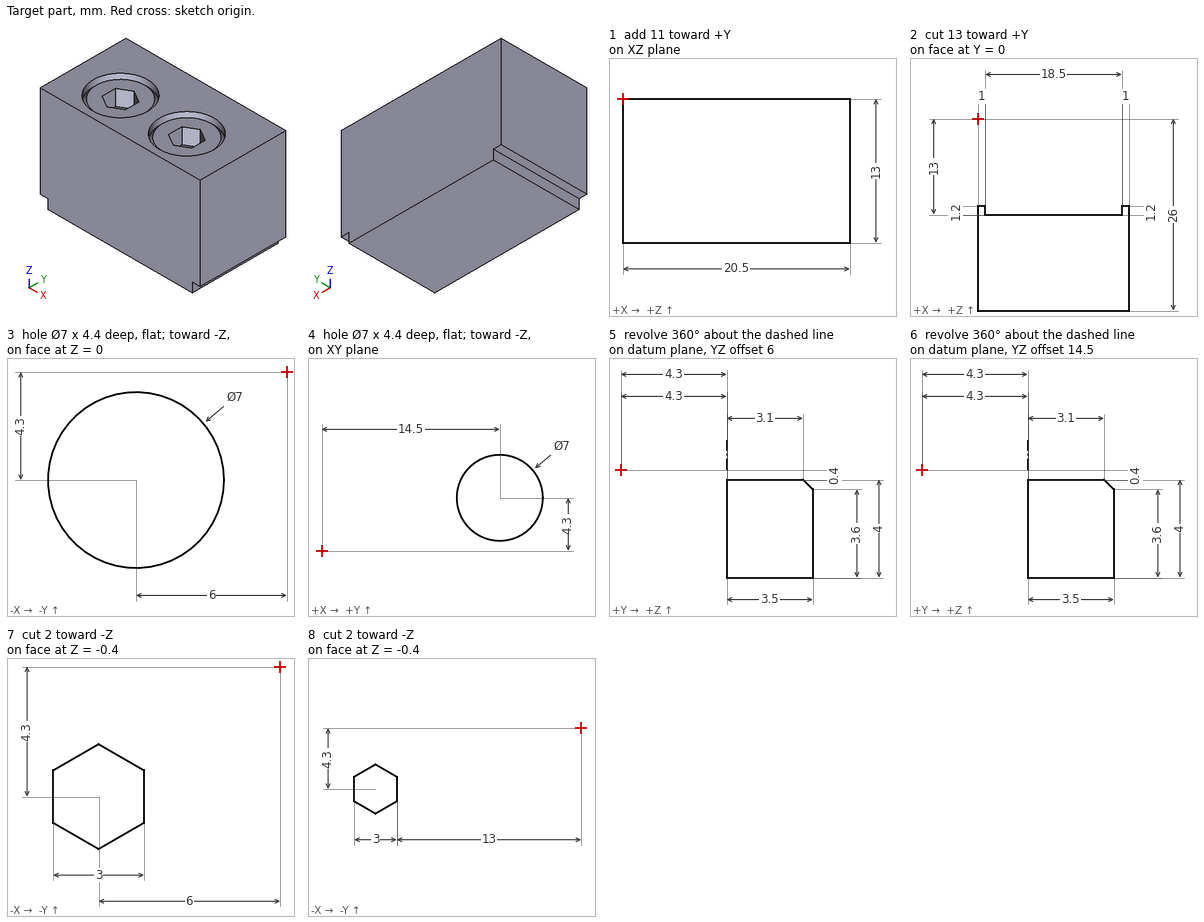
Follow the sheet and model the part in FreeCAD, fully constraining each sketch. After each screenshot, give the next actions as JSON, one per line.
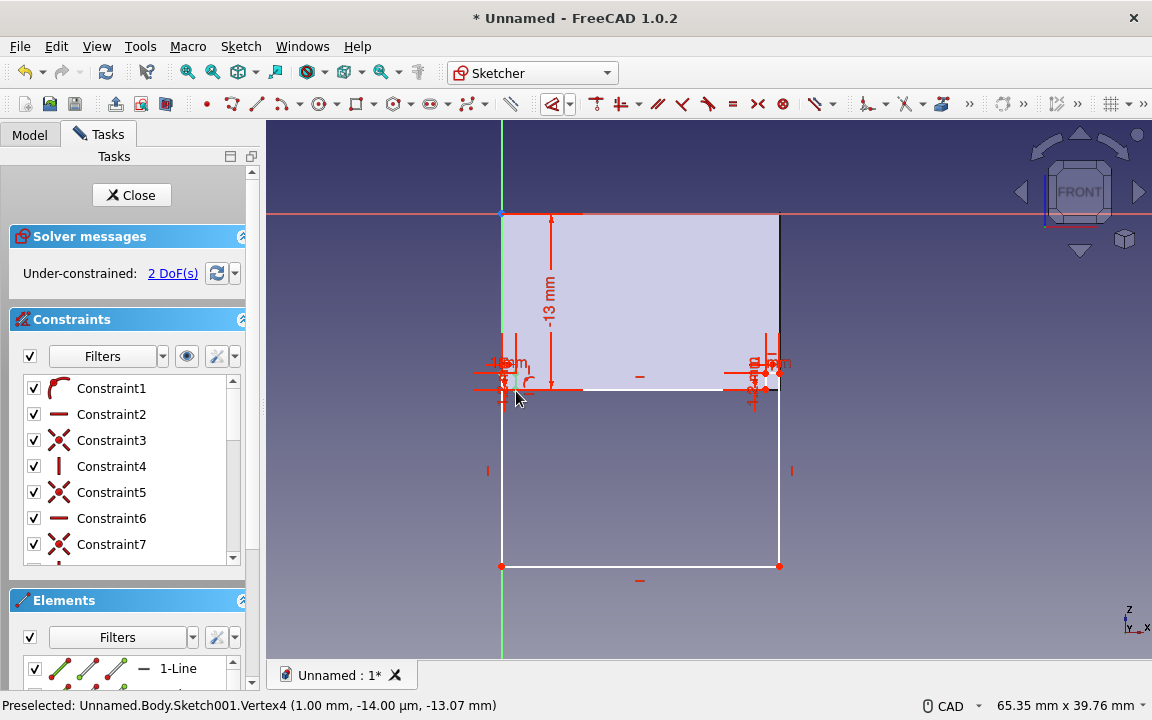
{"action": "left_click", "coordinate": [779, 567]}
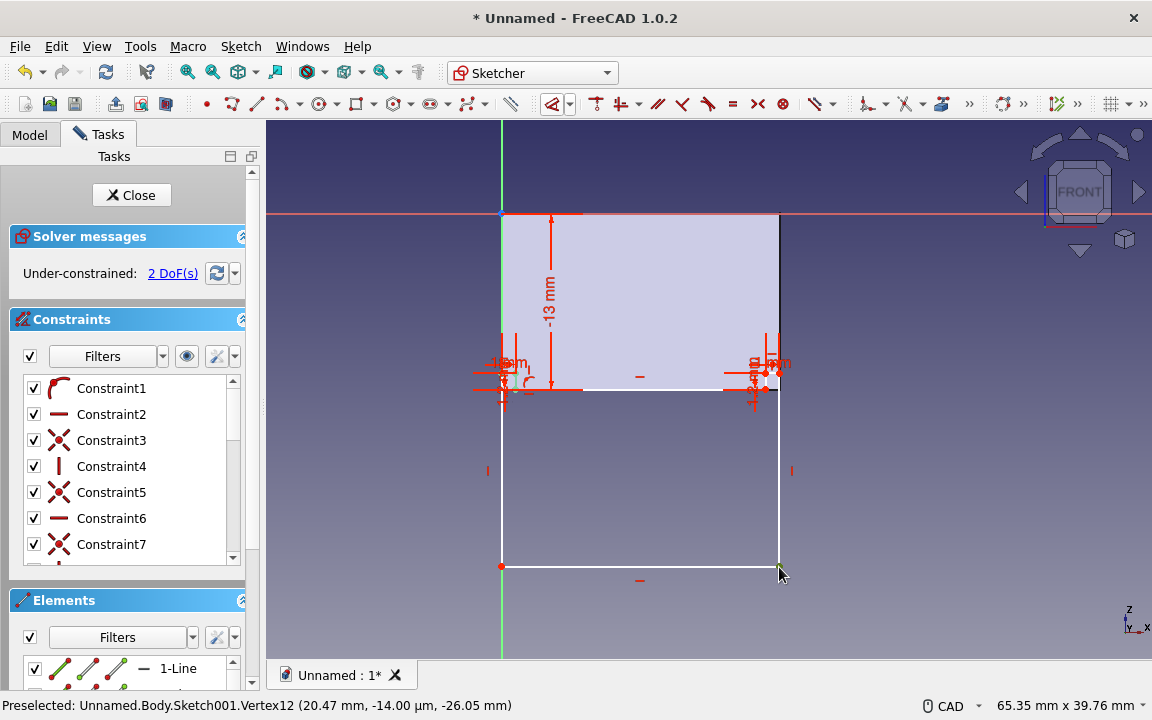
{"action": "left_click", "coordinate": [570, 104]}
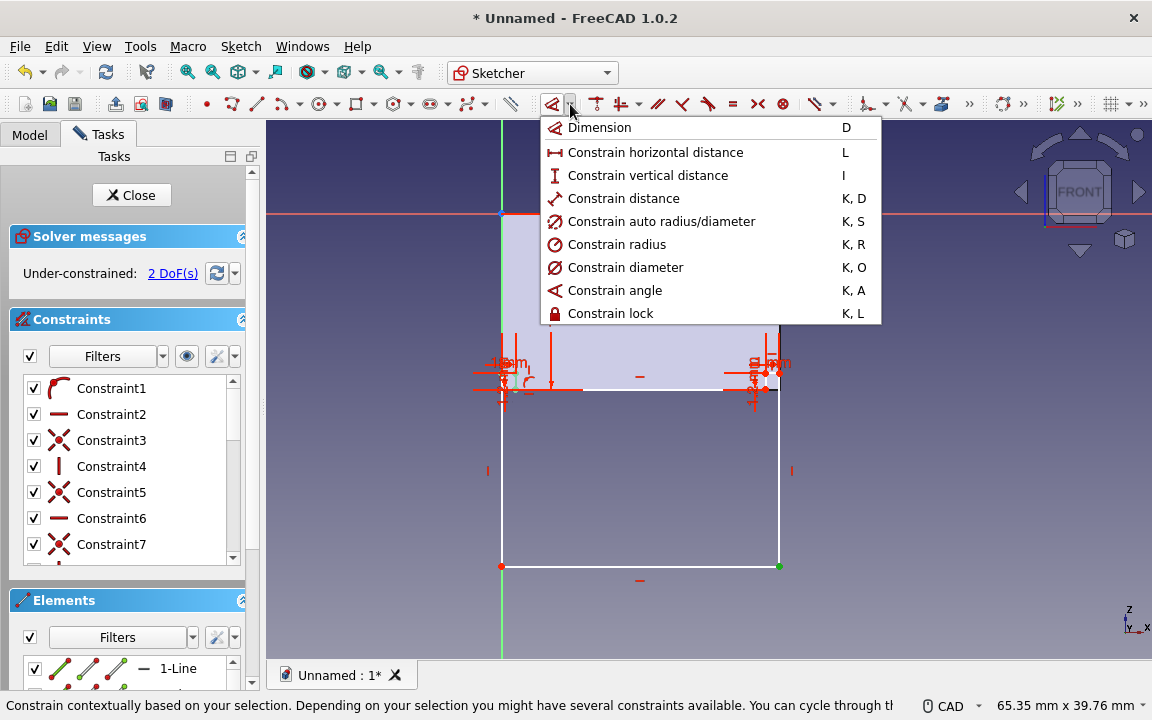
{"action": "left_click", "coordinate": [711, 176]}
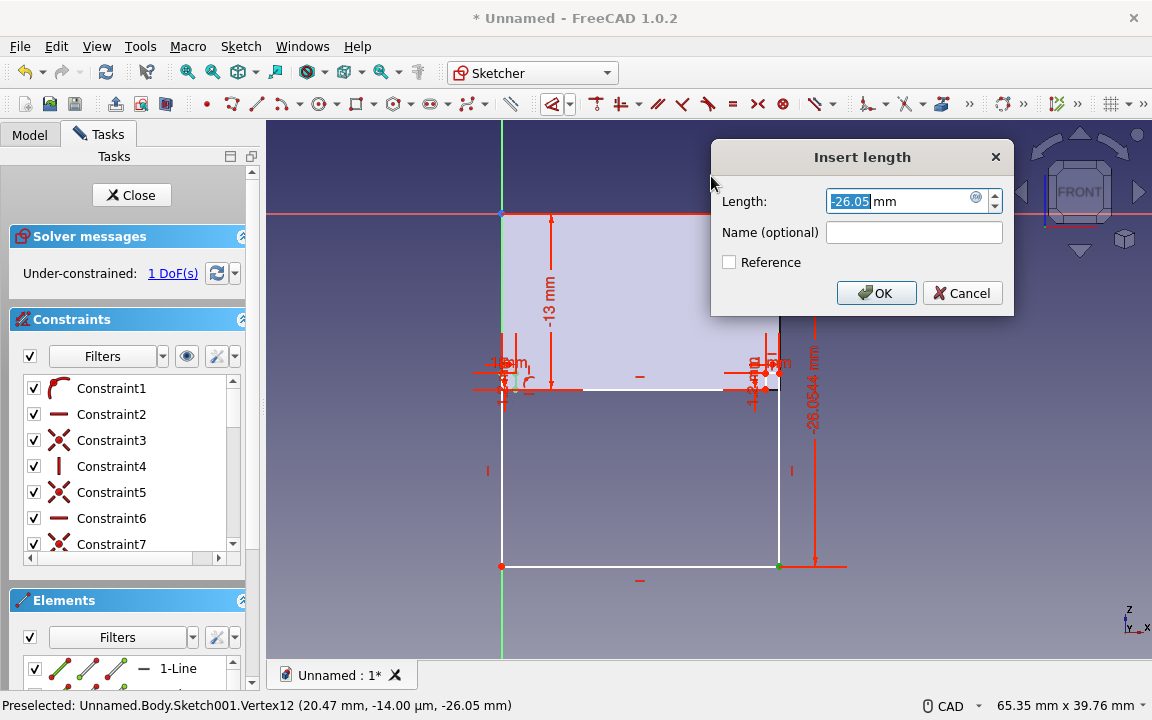
{"action": "type", "text": "-26"}
{"action": "key", "text": "Return"}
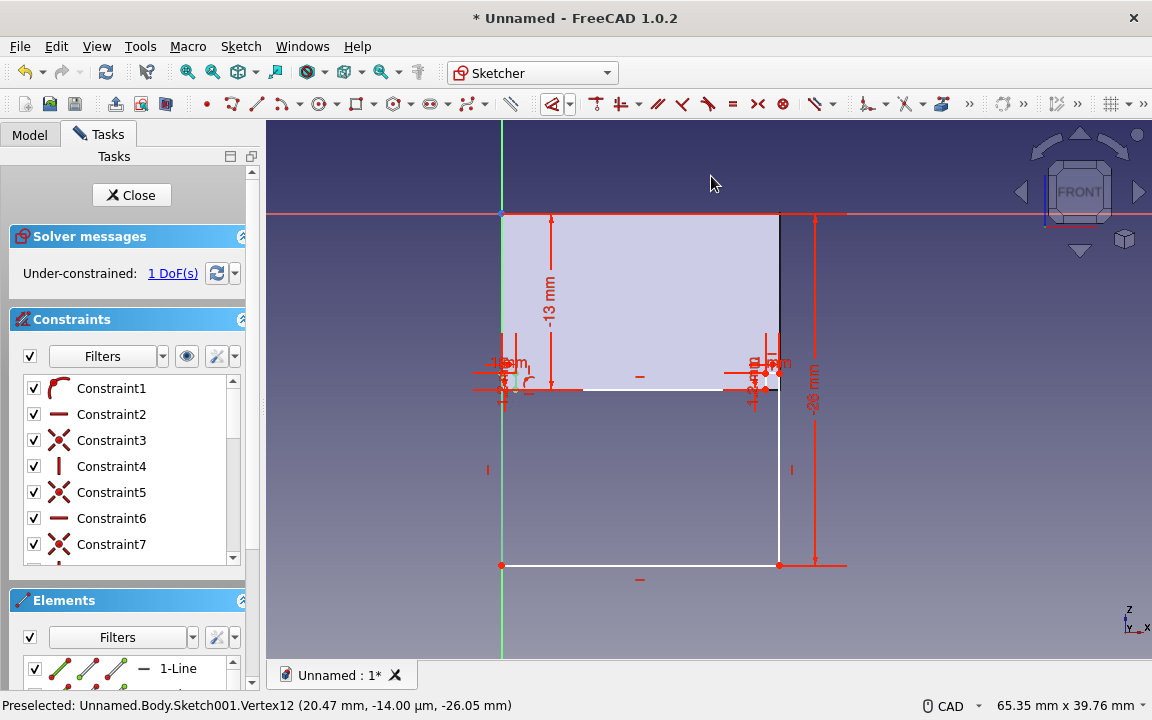
{"action": "left_click", "coordinate": [591, 390]}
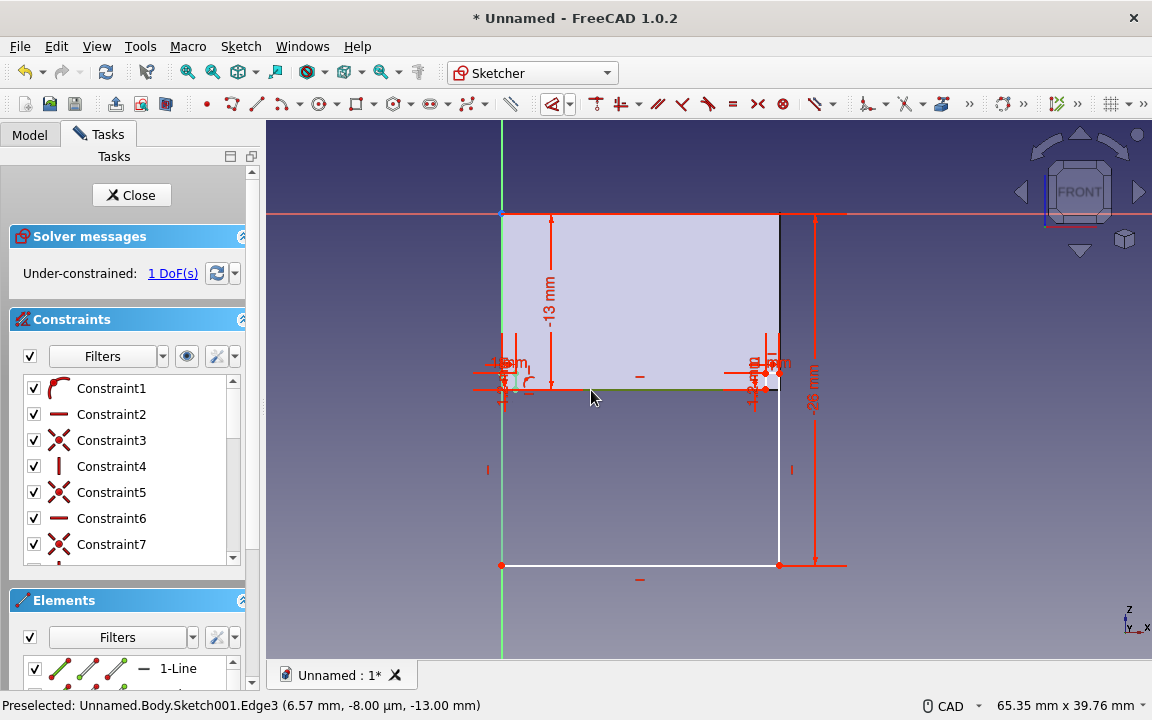
{"action": "key", "text": "l"}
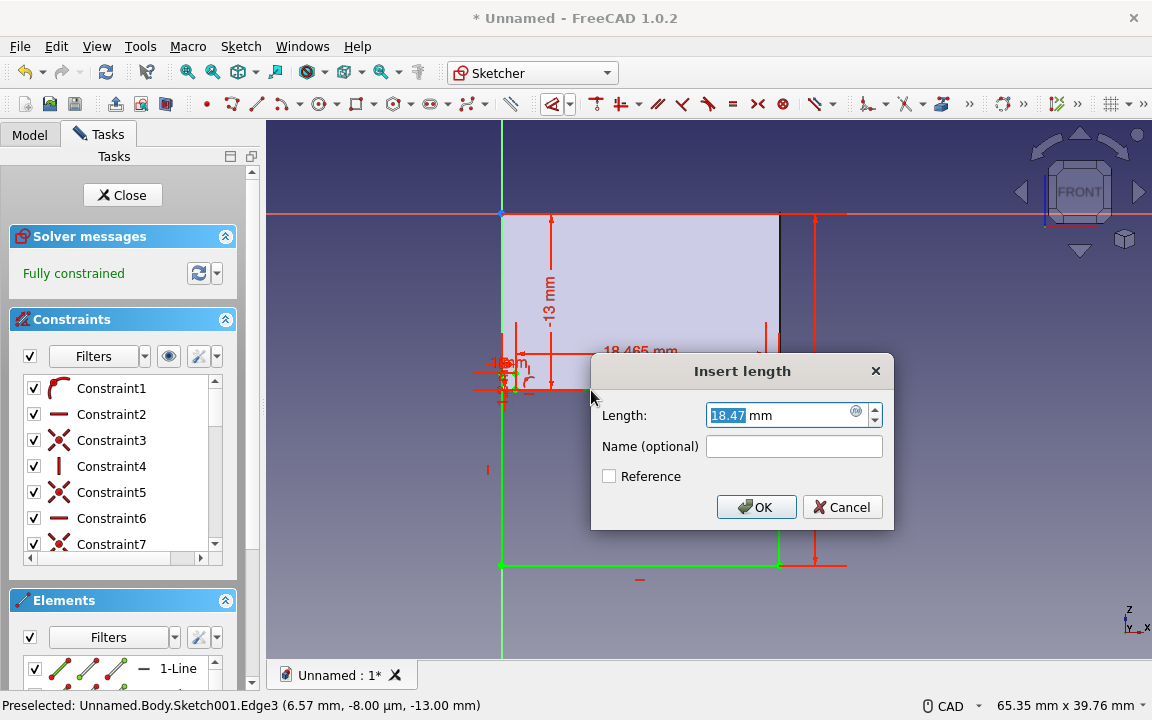
{"action": "type", "text": "18.5"}
{"action": "key", "text": "Return"}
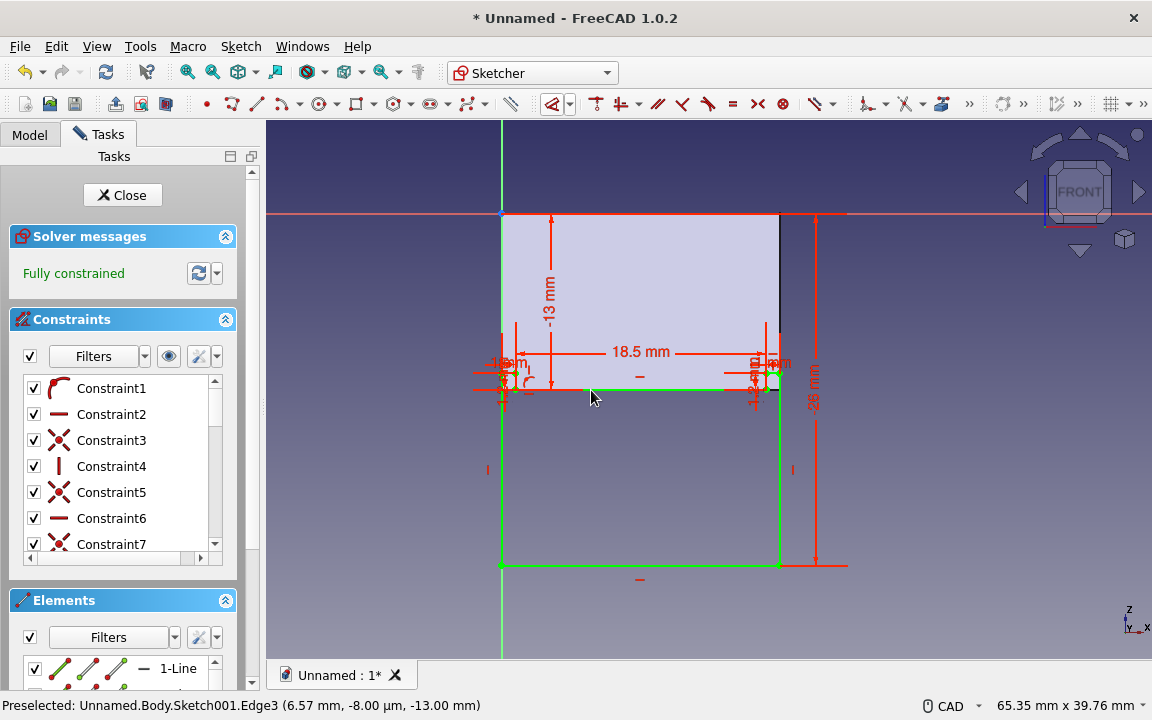
{"action": "left_click", "coordinate": [123, 195]}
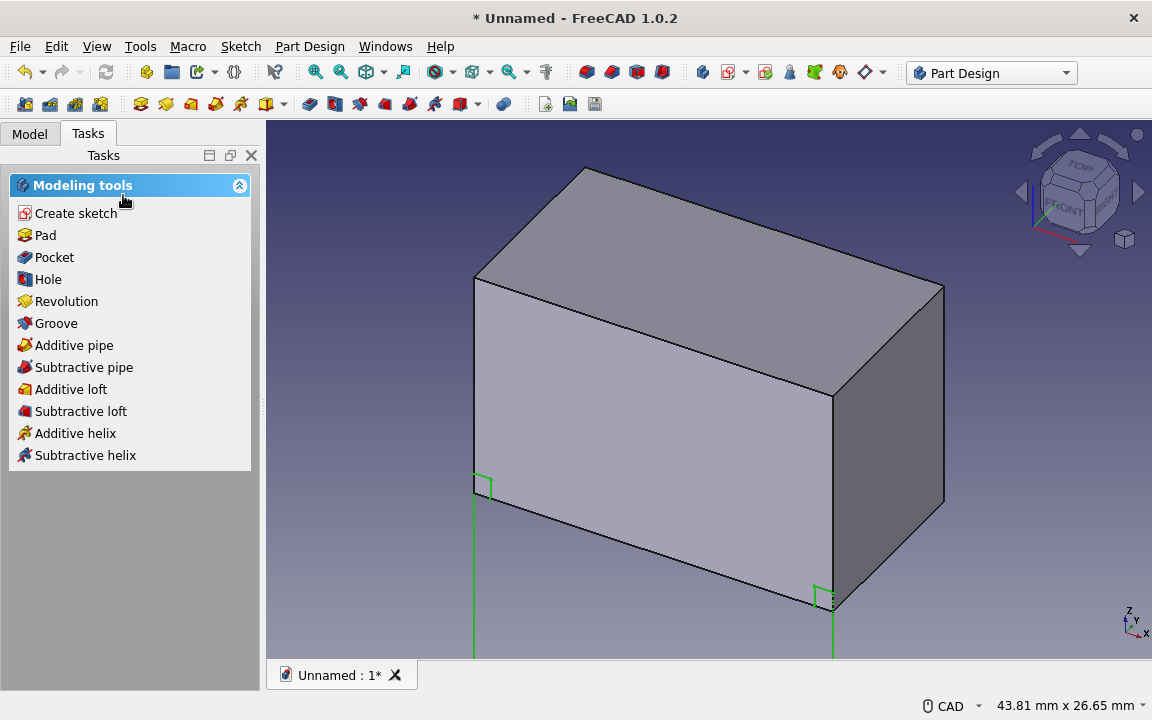
{"action": "left_click", "coordinate": [310, 104]}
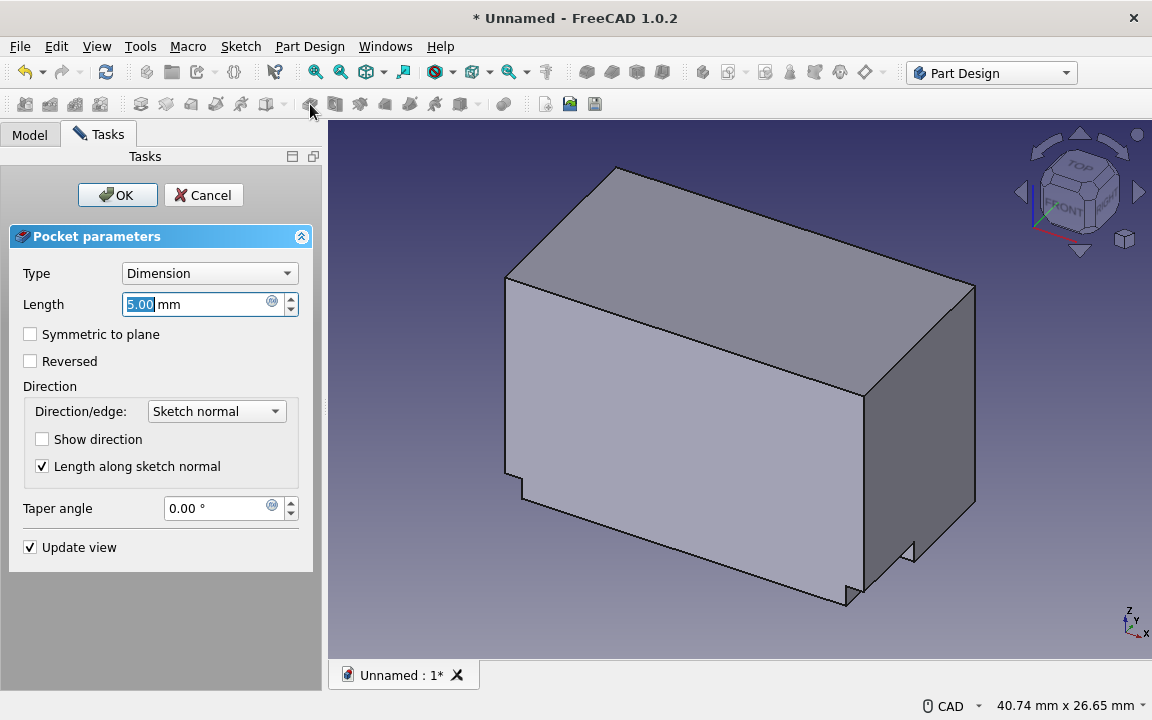
{"action": "type", "text": "13"}
{"action": "key", "text": "Tab"}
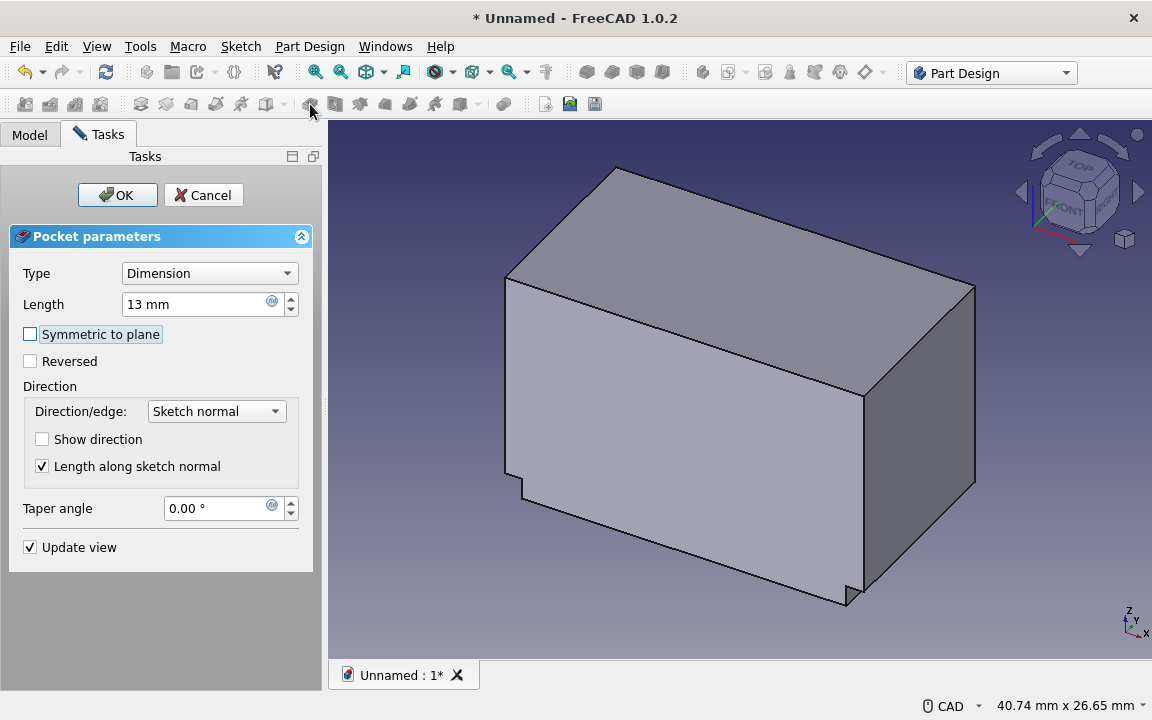
{"action": "left_click", "coordinate": [118, 195]}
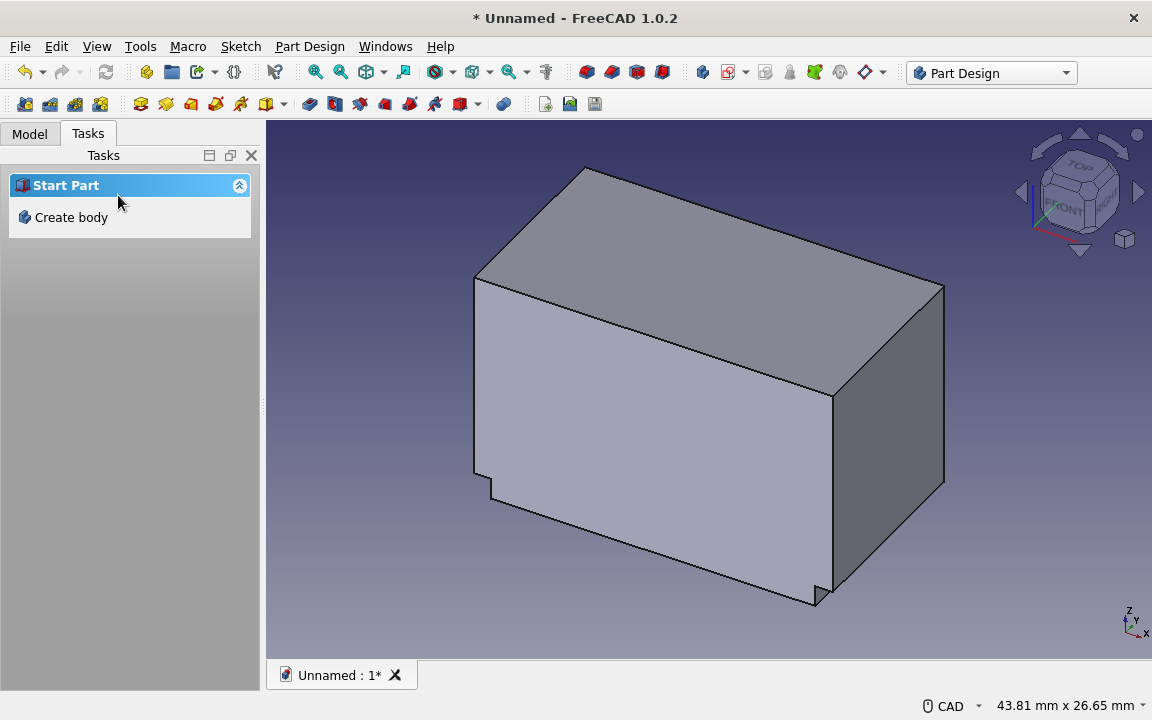
{"action": "left_click", "coordinate": [760, 298]}